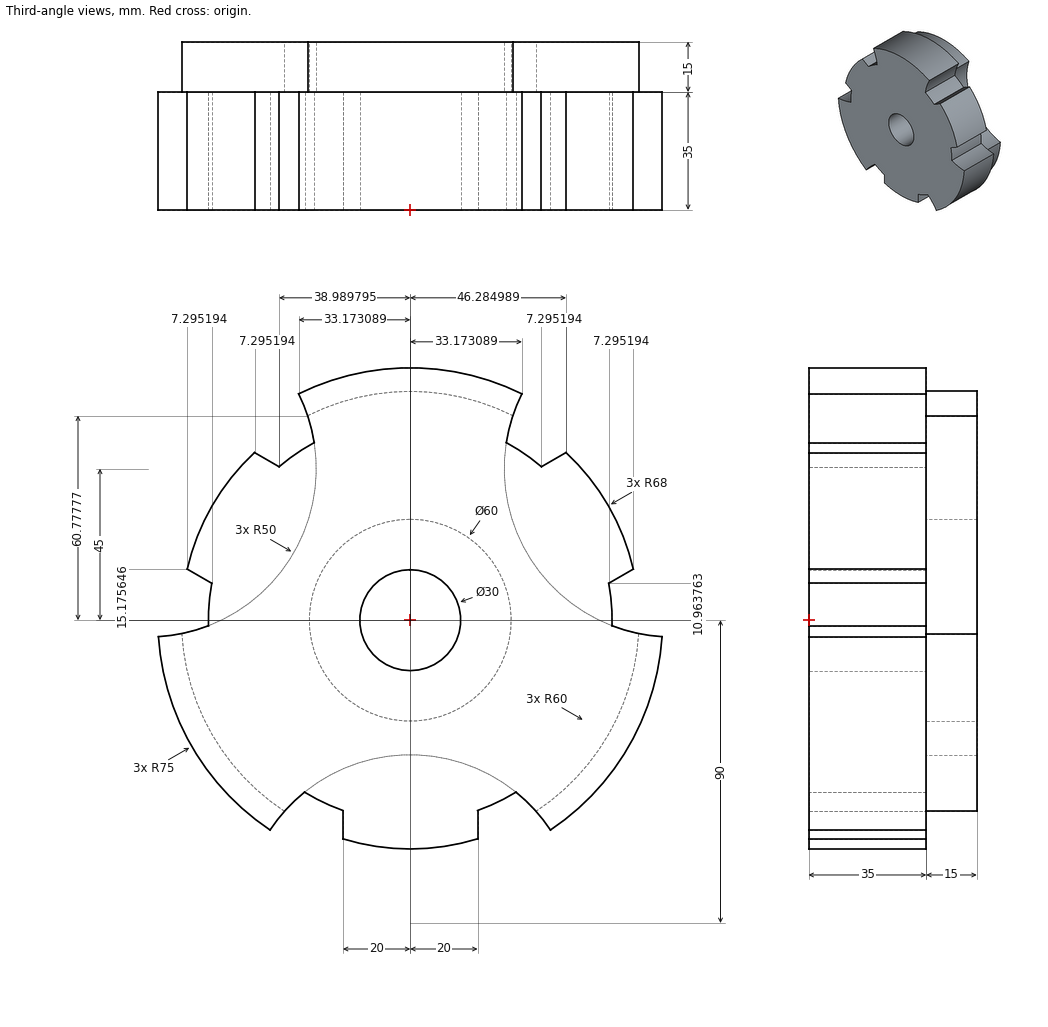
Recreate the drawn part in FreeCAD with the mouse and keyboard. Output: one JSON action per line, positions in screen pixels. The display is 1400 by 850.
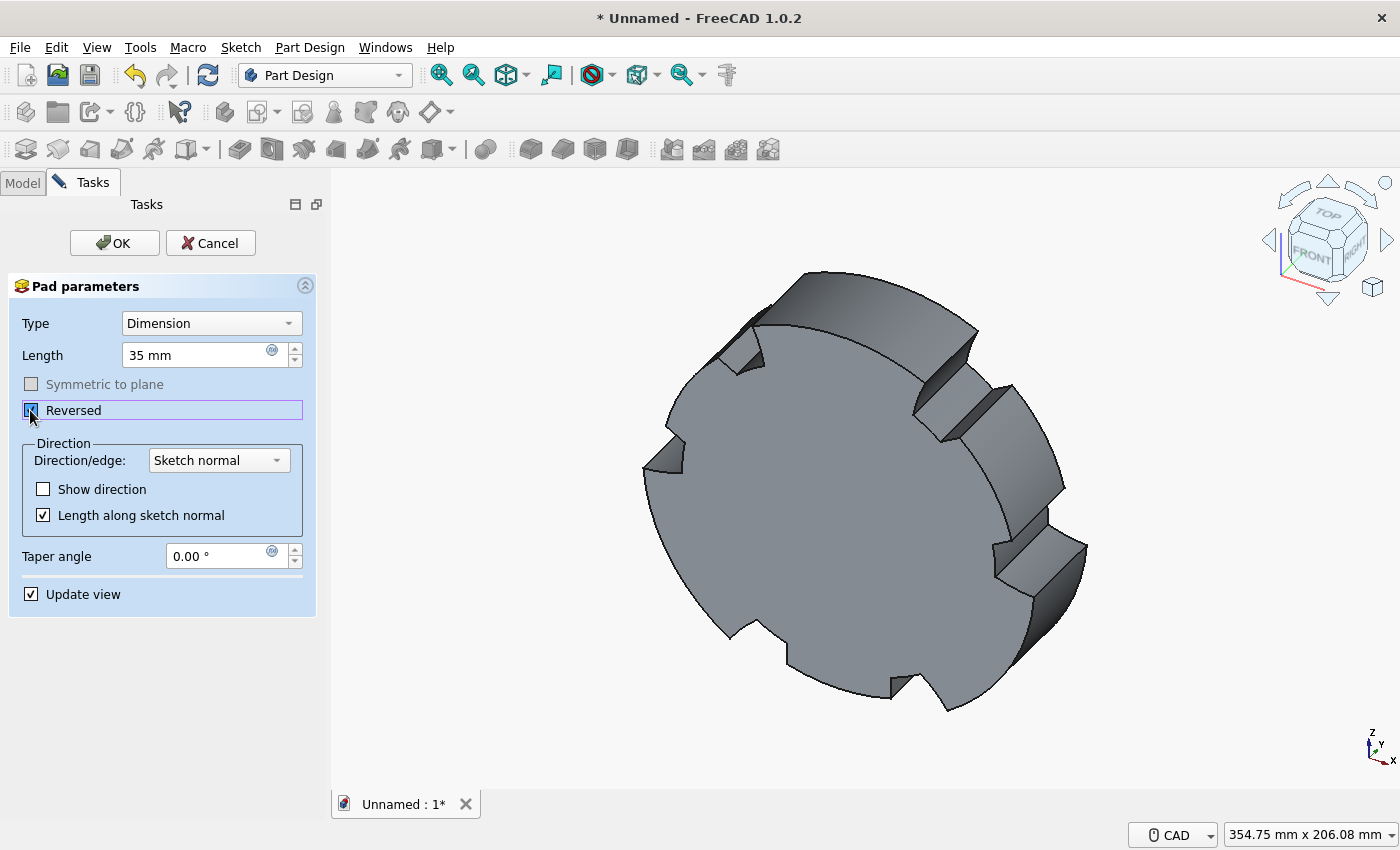
{"action": "left_click", "coordinate": [115, 243]}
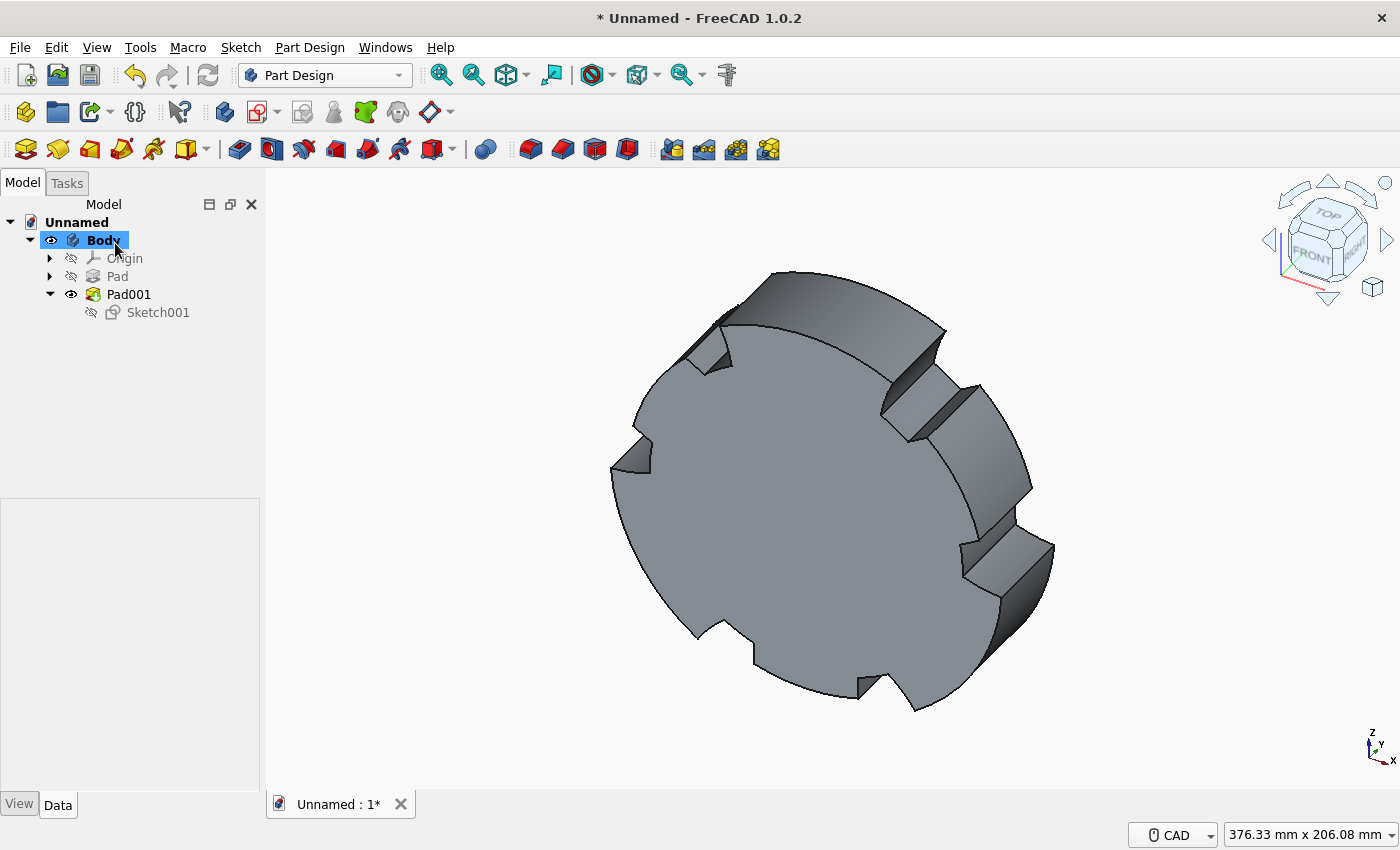
{"action": "key", "text": "4"}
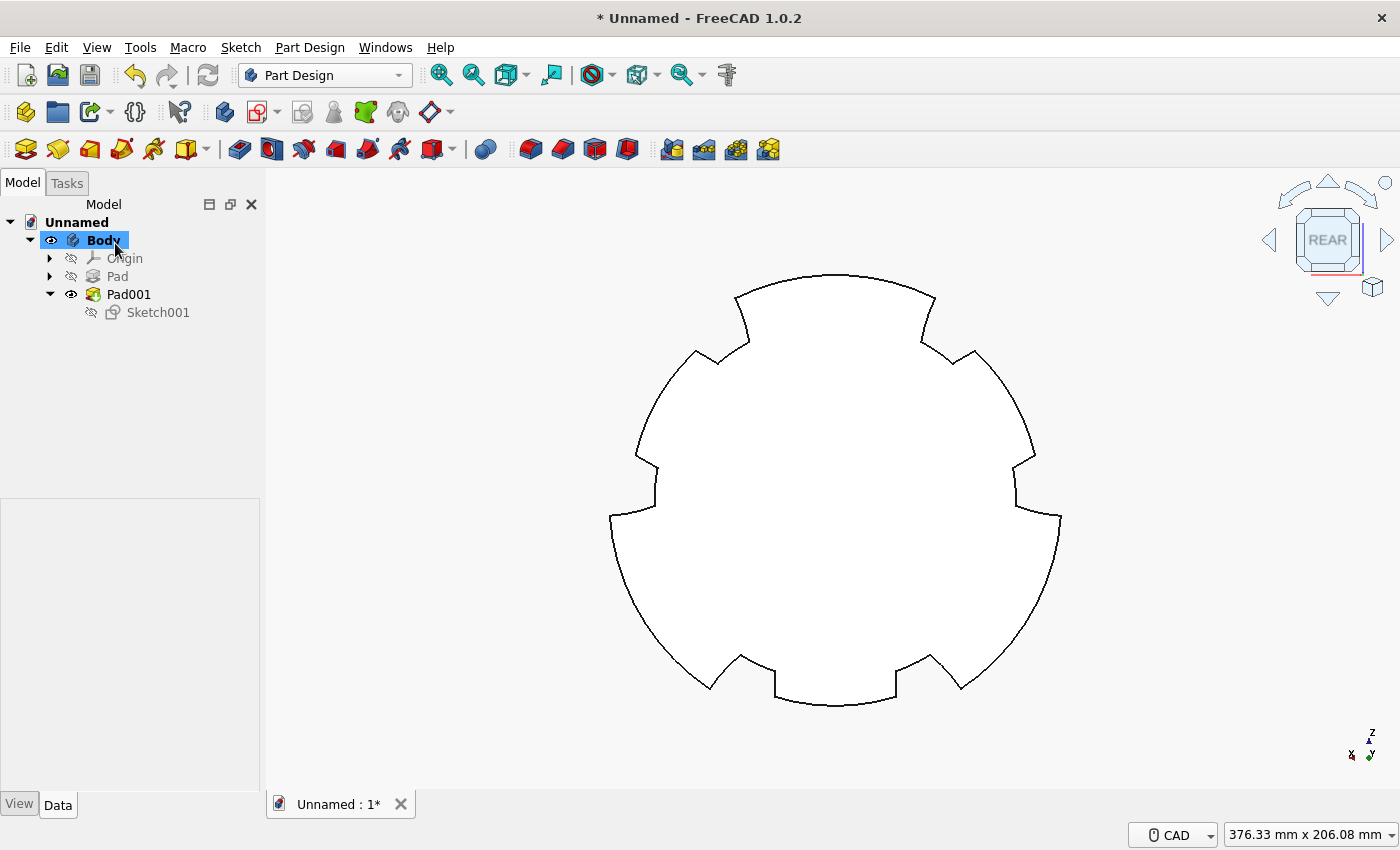
{"action": "left_click", "coordinate": [835, 489]}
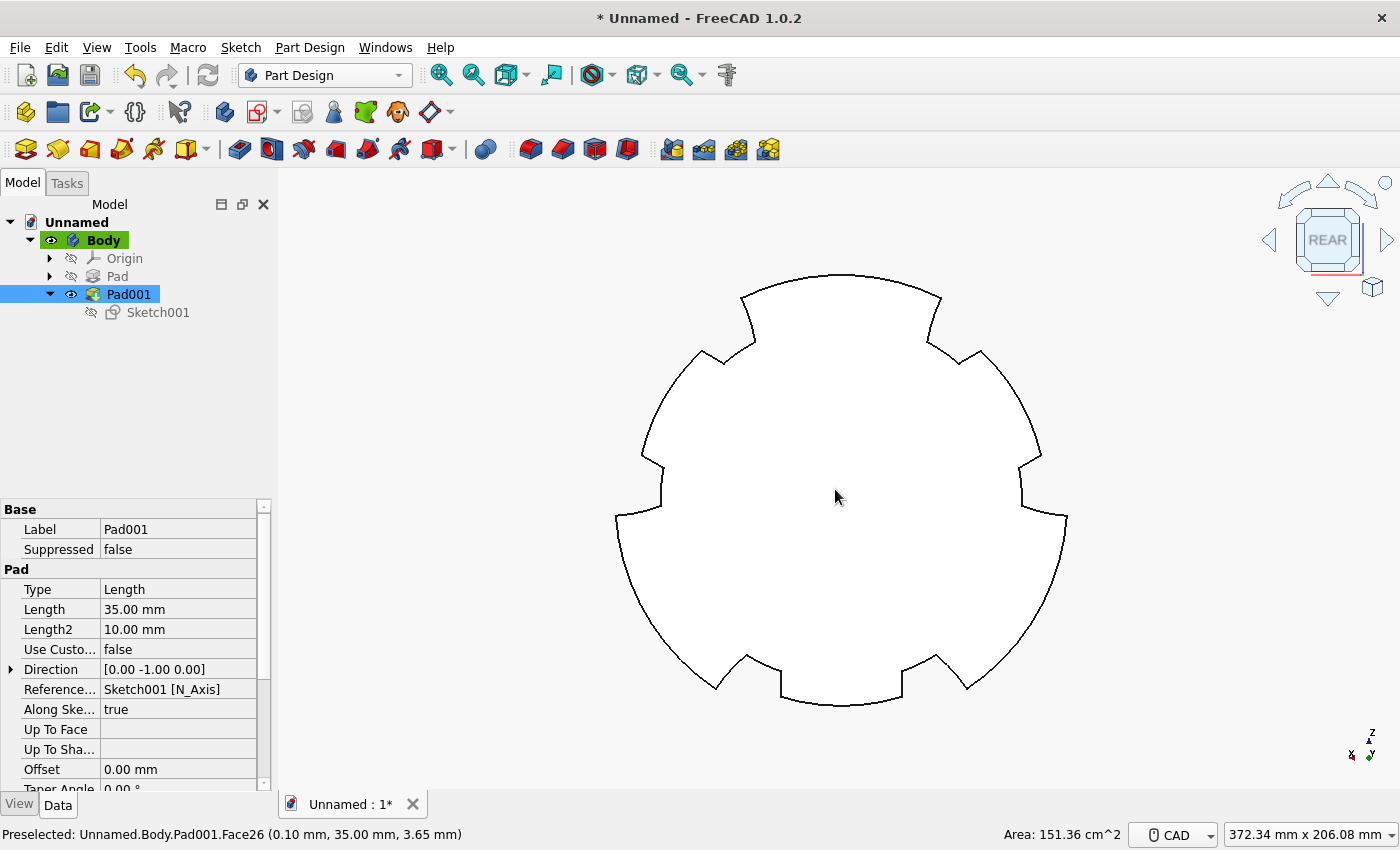
{"action": "left_click", "coordinate": [258, 112]}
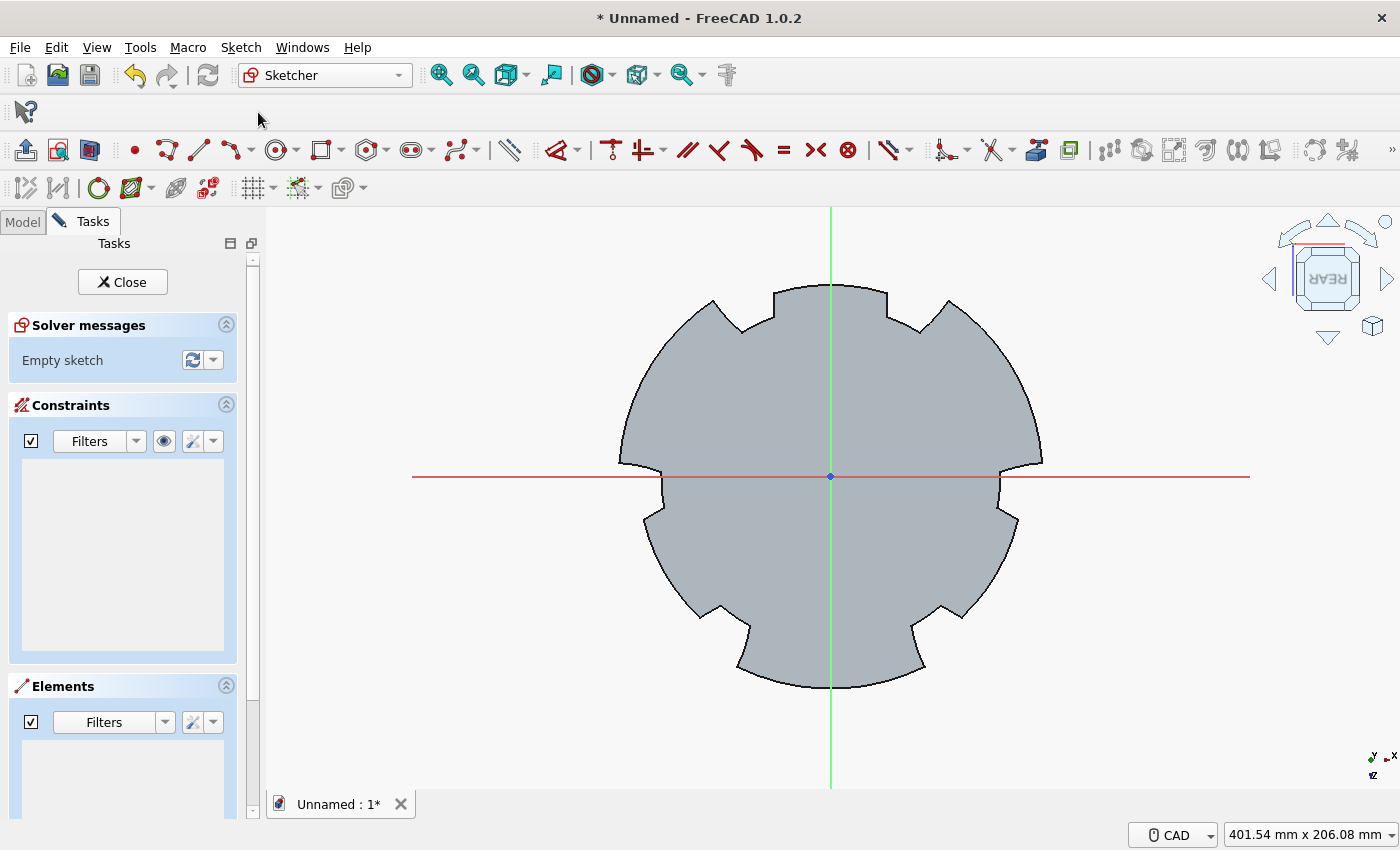
{"action": "left_click", "coordinate": [232, 150]}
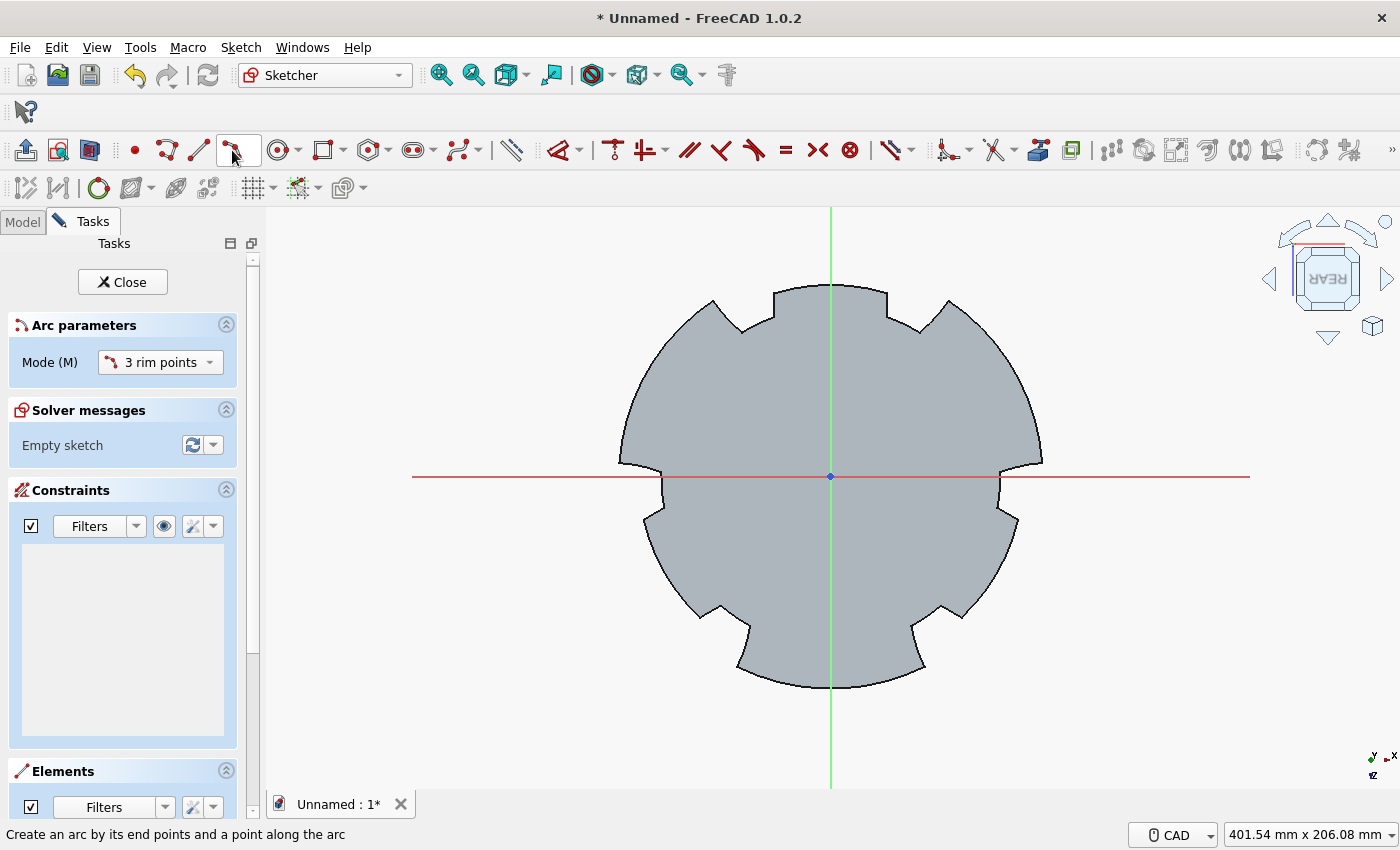
{"action": "left_click", "coordinate": [725, 316]}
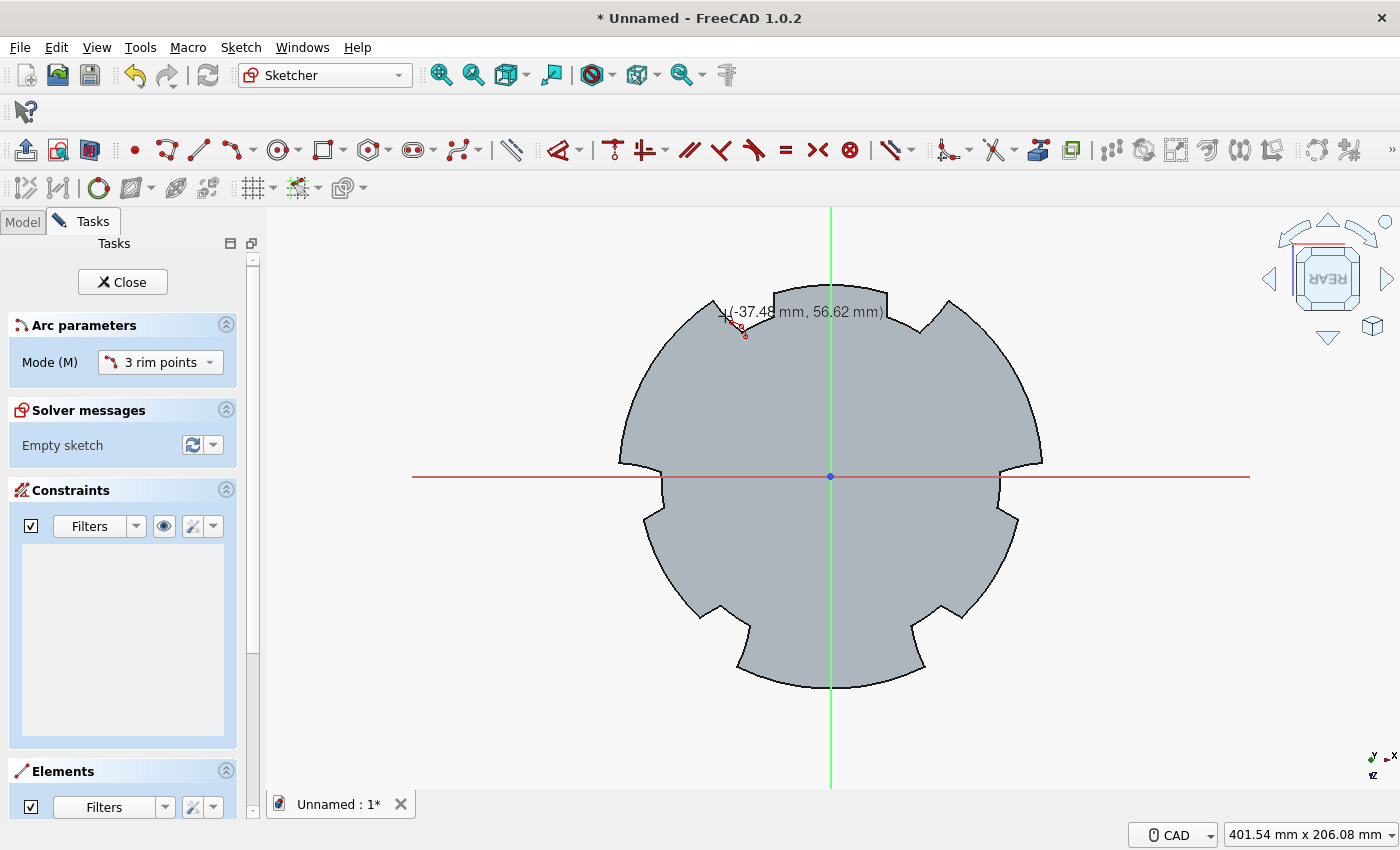
{"action": "scroll", "coordinate": [639, 466], "scroll_direction": "up", "scroll_amount": 2}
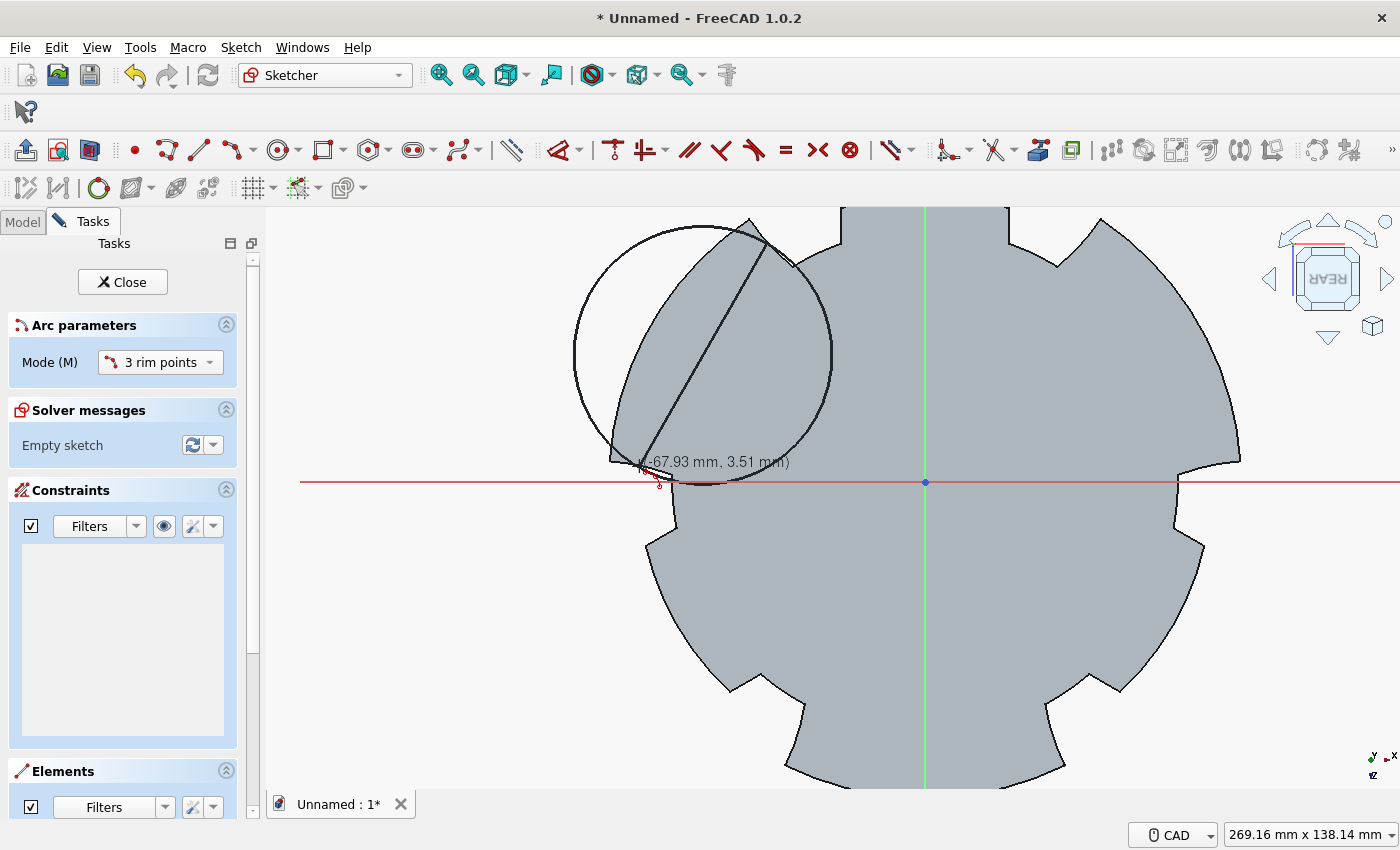
{"action": "left_click", "coordinate": [639, 465]}
{"action": "left_click", "coordinate": [677, 339]}